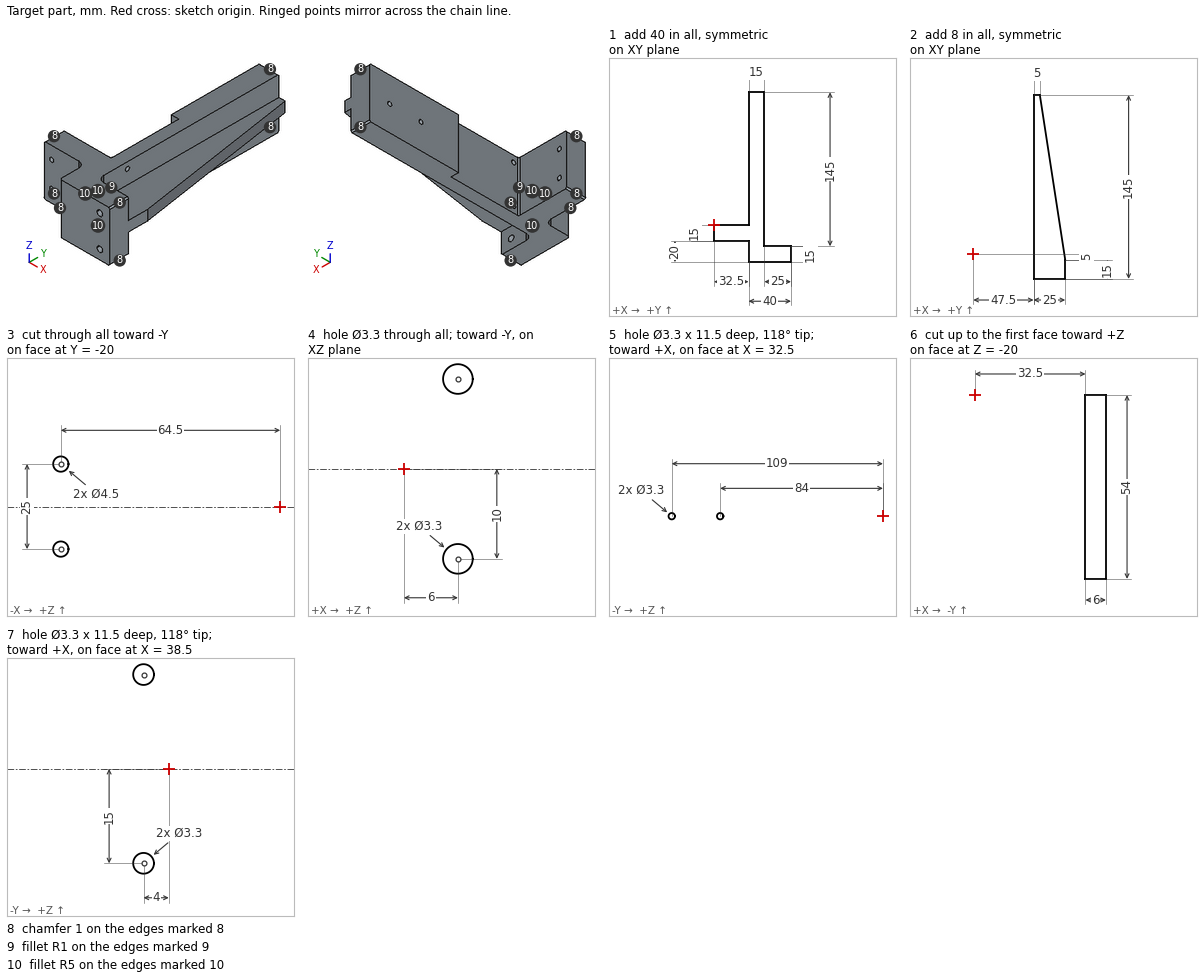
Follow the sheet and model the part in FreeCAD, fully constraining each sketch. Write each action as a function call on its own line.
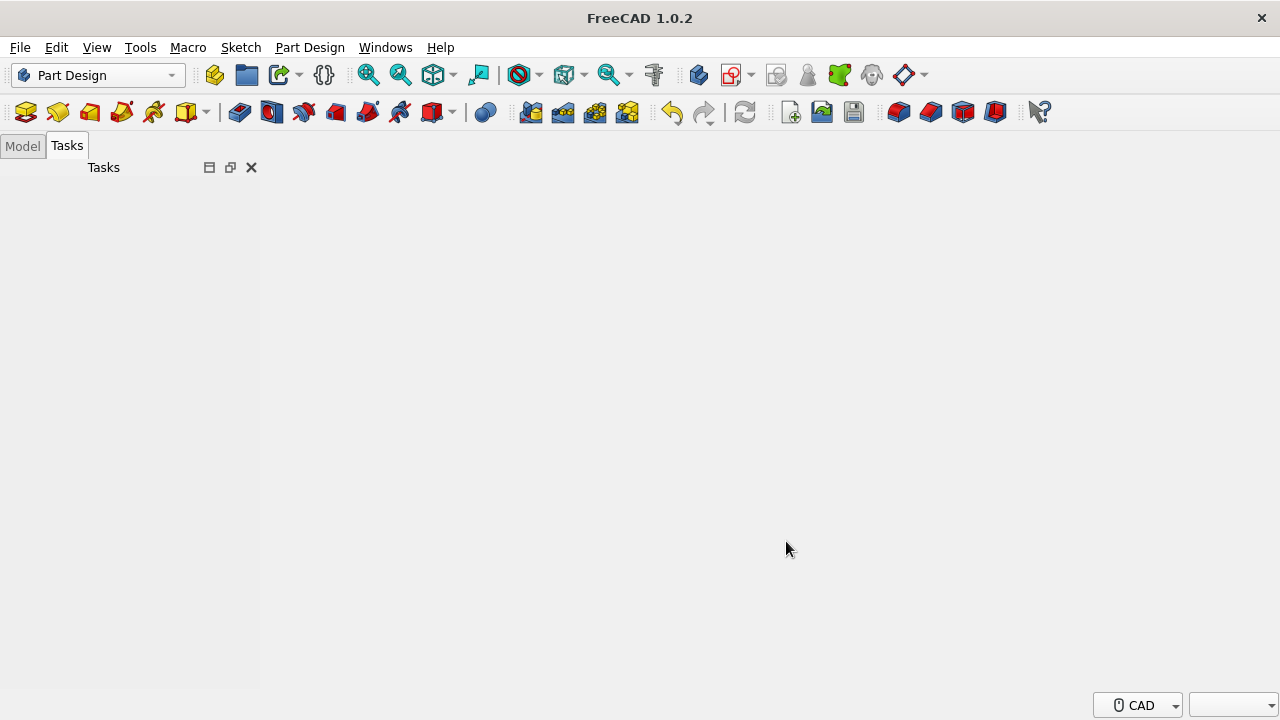
click(790, 112)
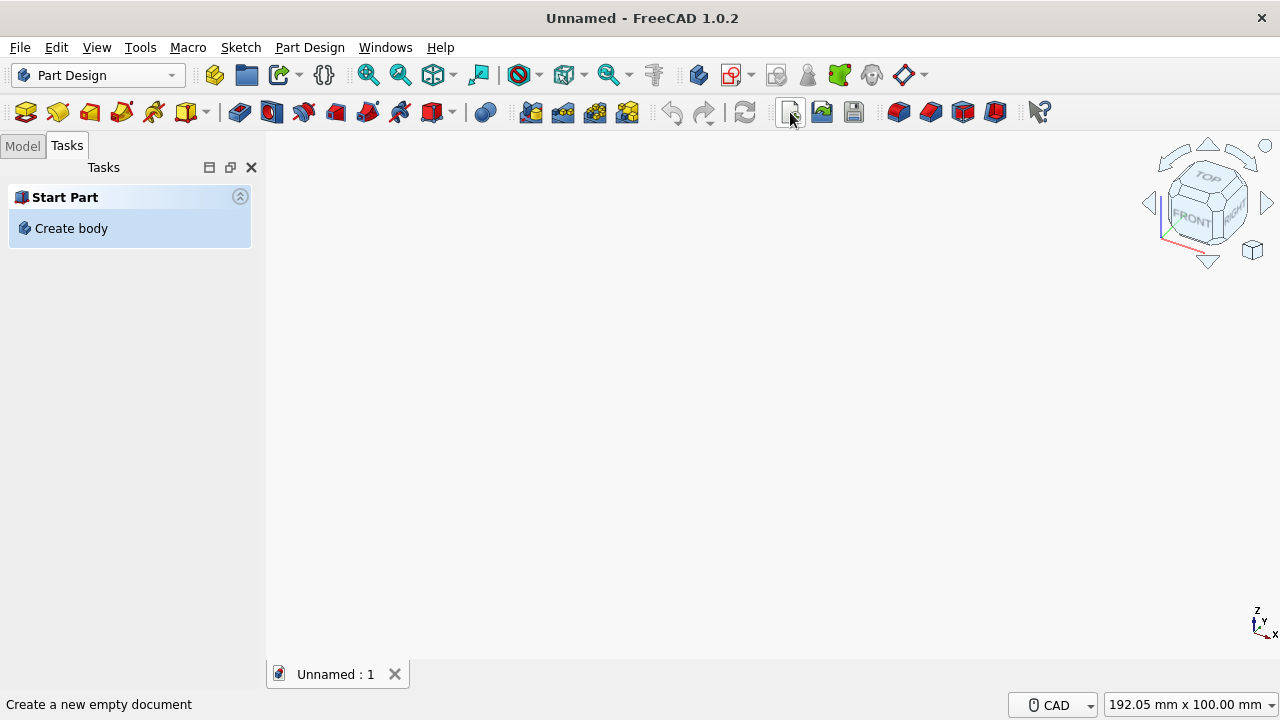
click(732, 76)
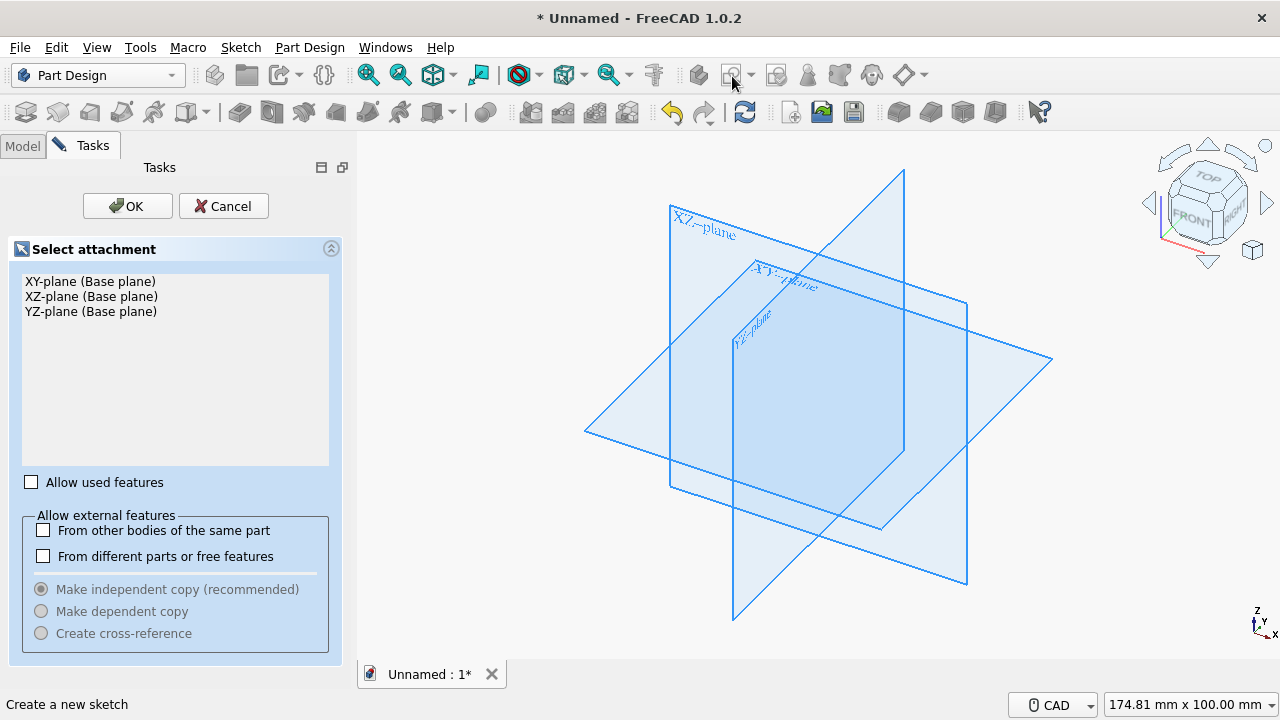
click(82, 282)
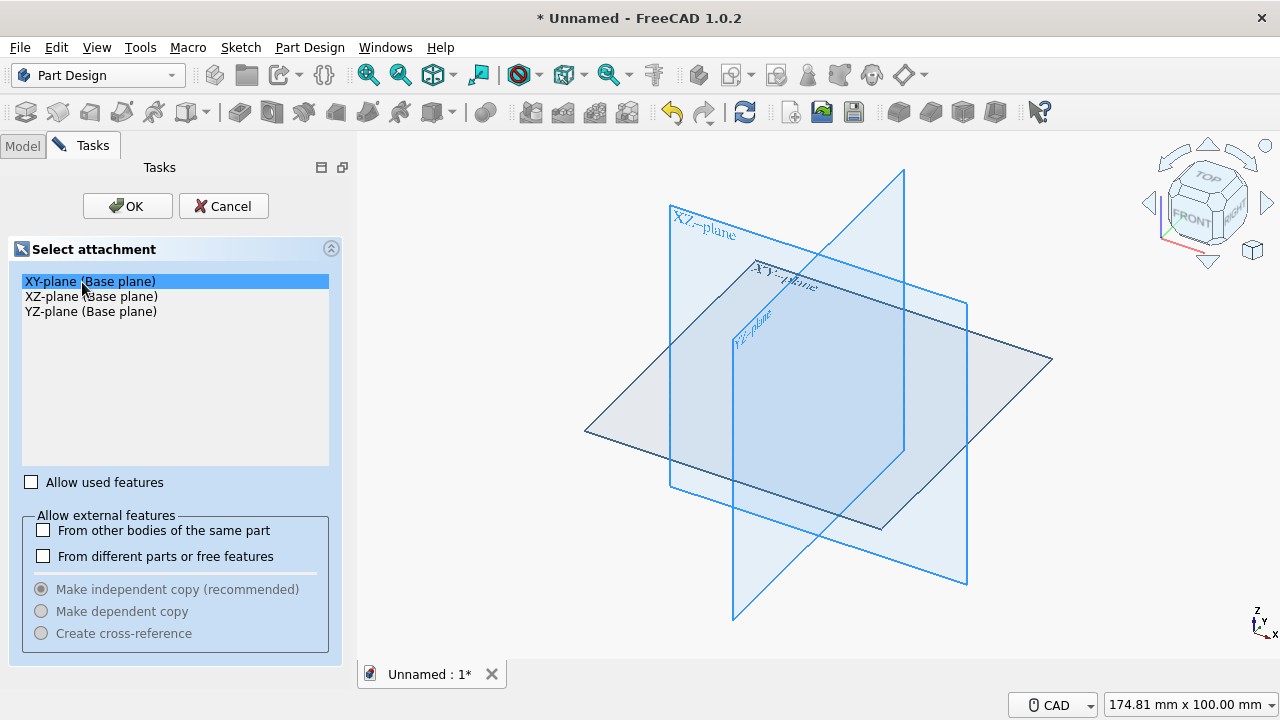
click(128, 206)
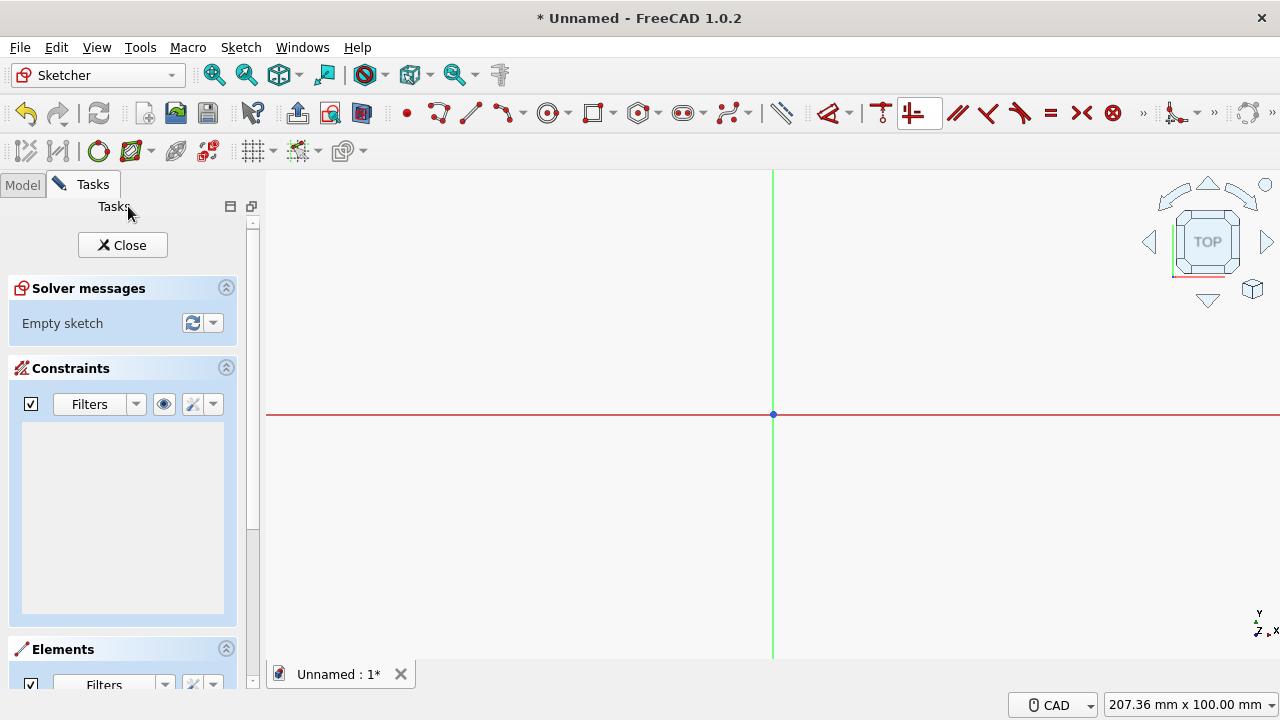
scroll(561, 543, down, 5)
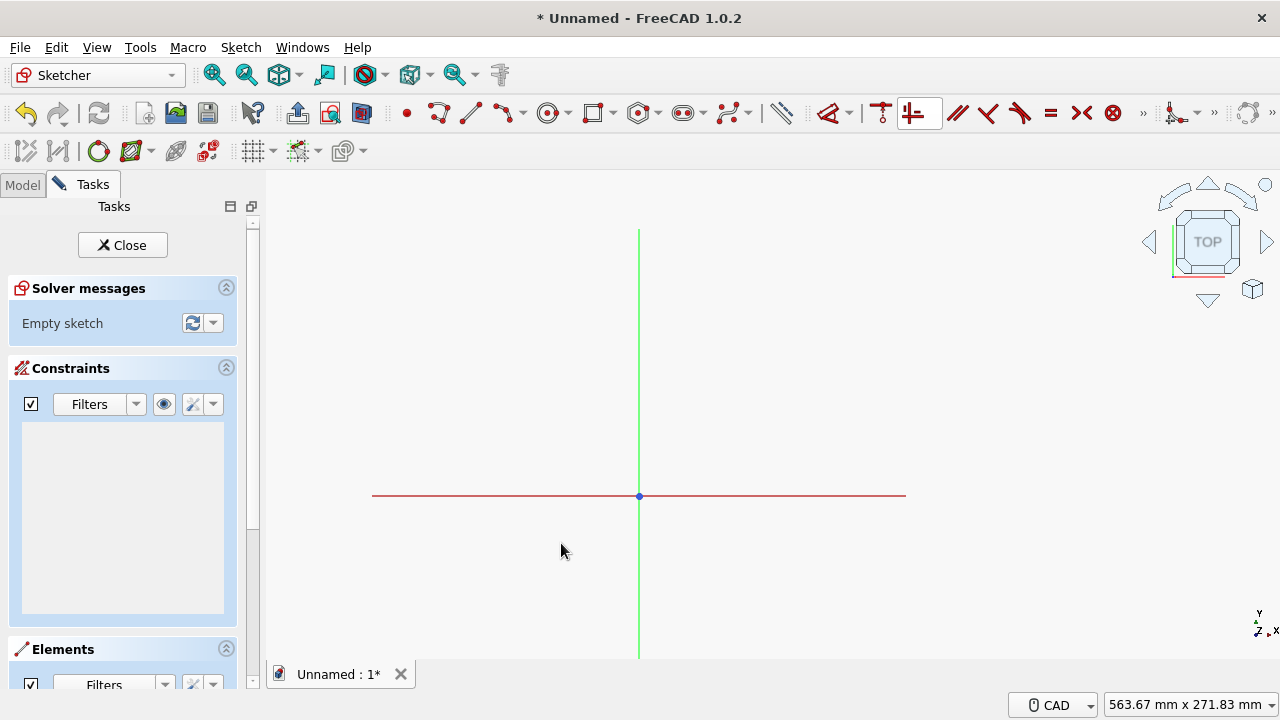
click(440, 114)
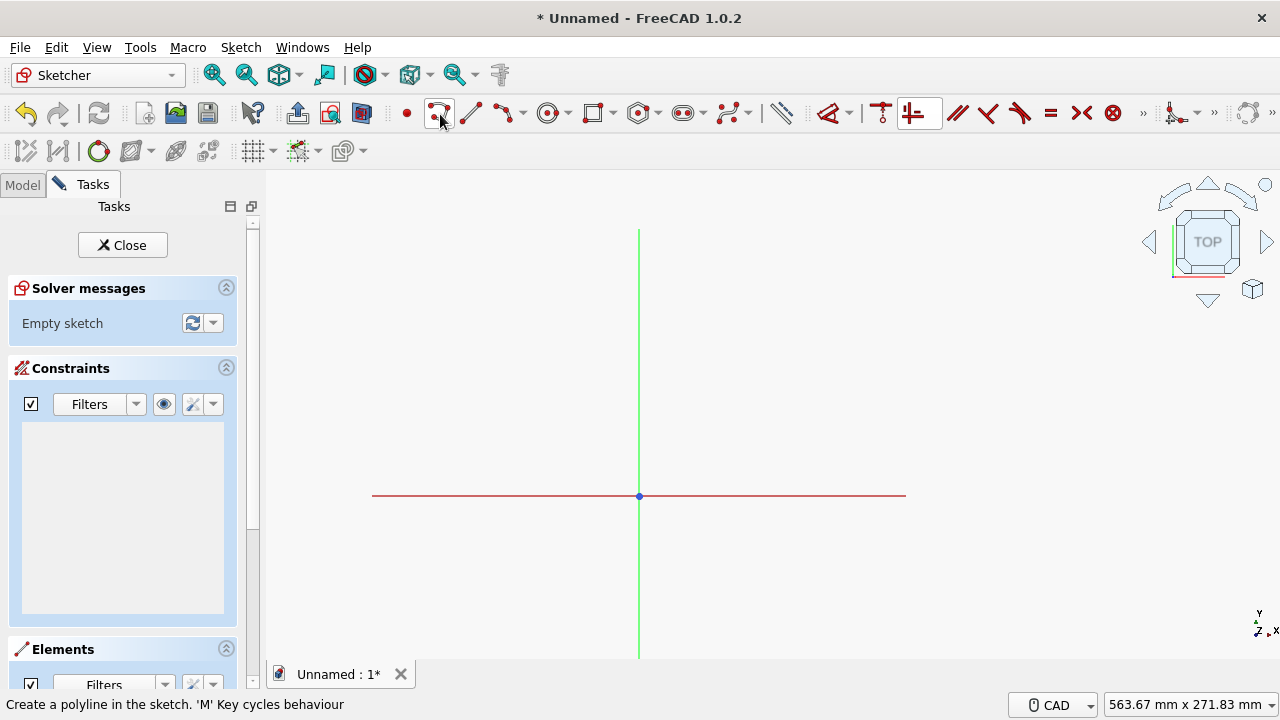
click(639, 496)
click(648, 523)
click(698, 523)
click(698, 559)
click(770, 559)
click(770, 532)
click(725, 532)
click(725, 271)
click(698, 271)
click(698, 487)
click(639, 496)
key(Escape)
key(Escape)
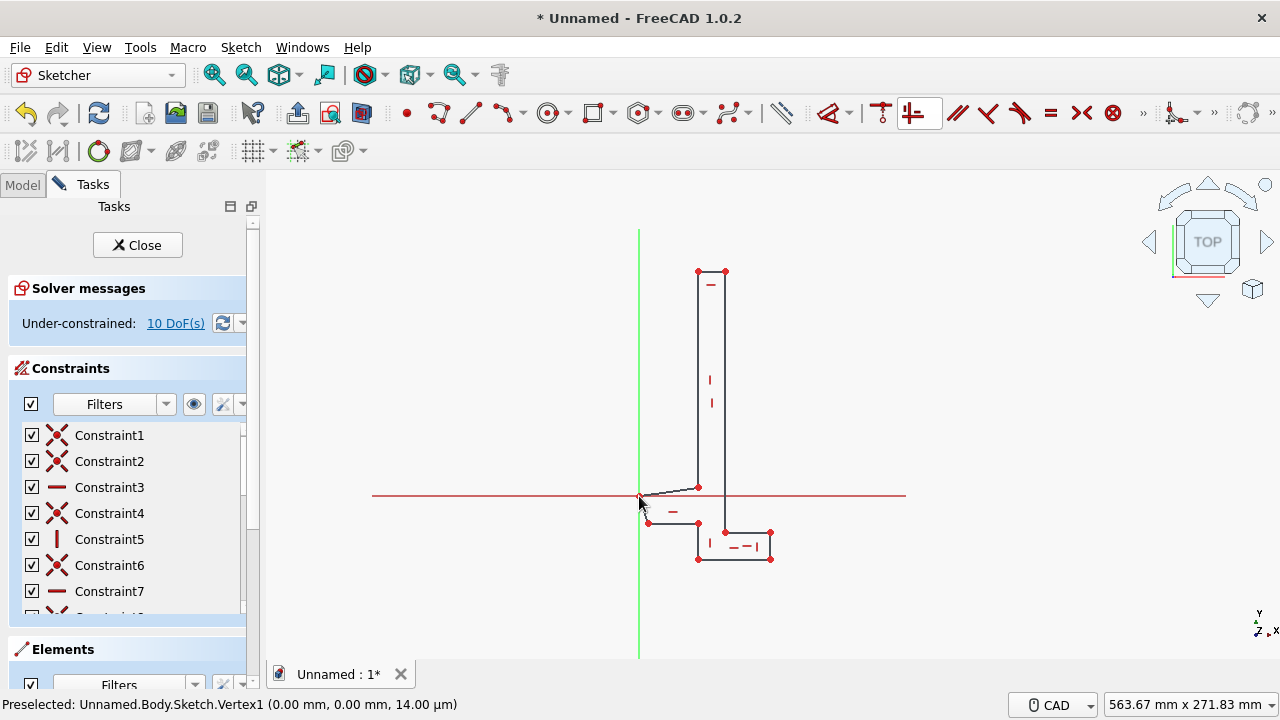
scroll(643, 507, up, 2)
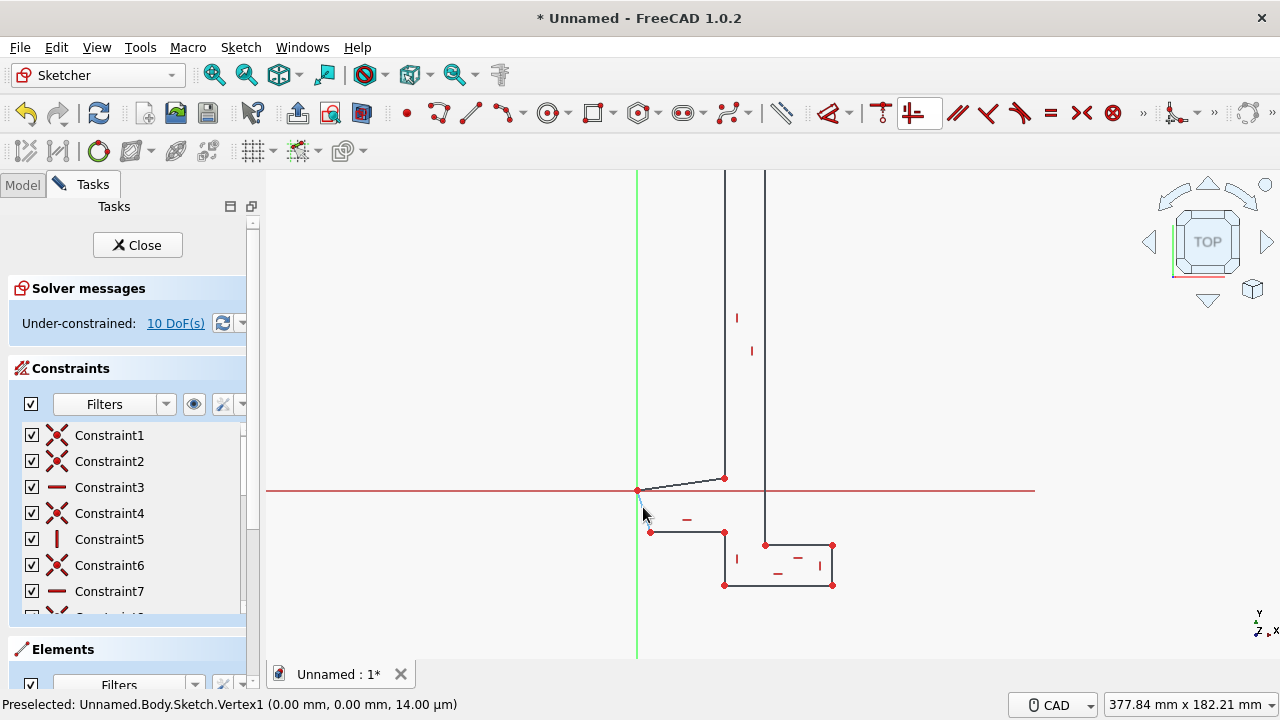
click(642, 507)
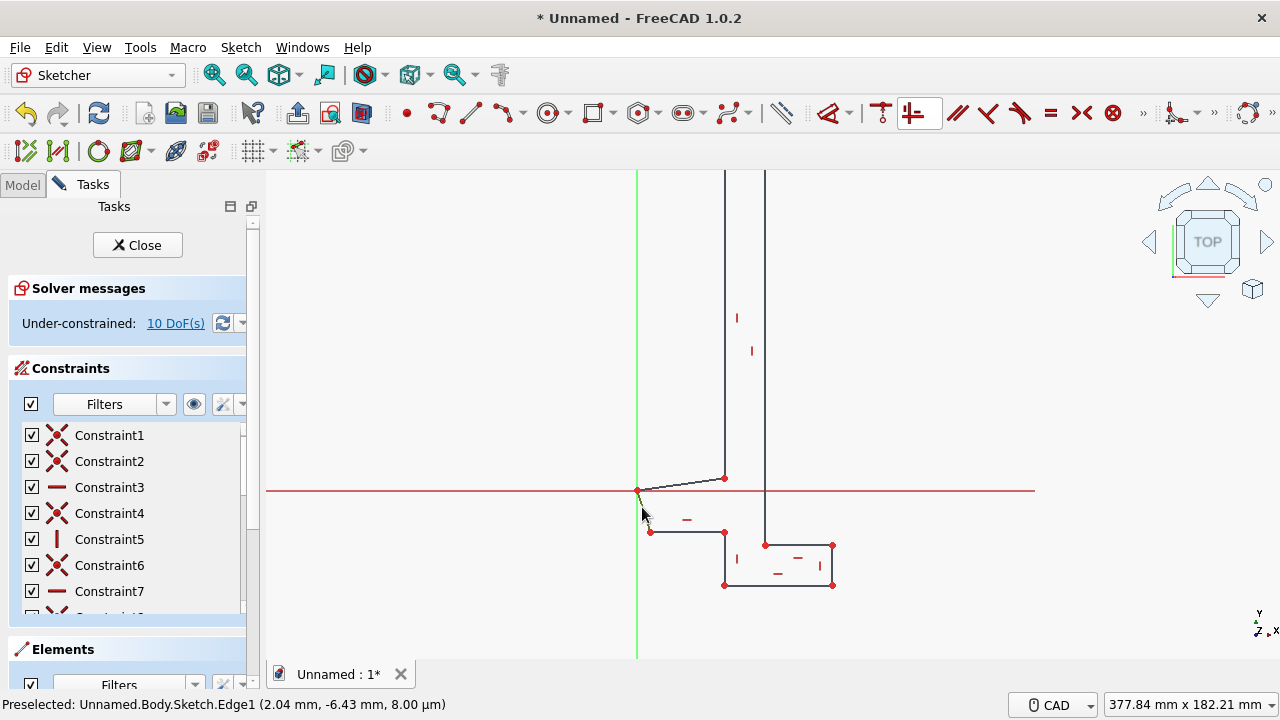
key(v)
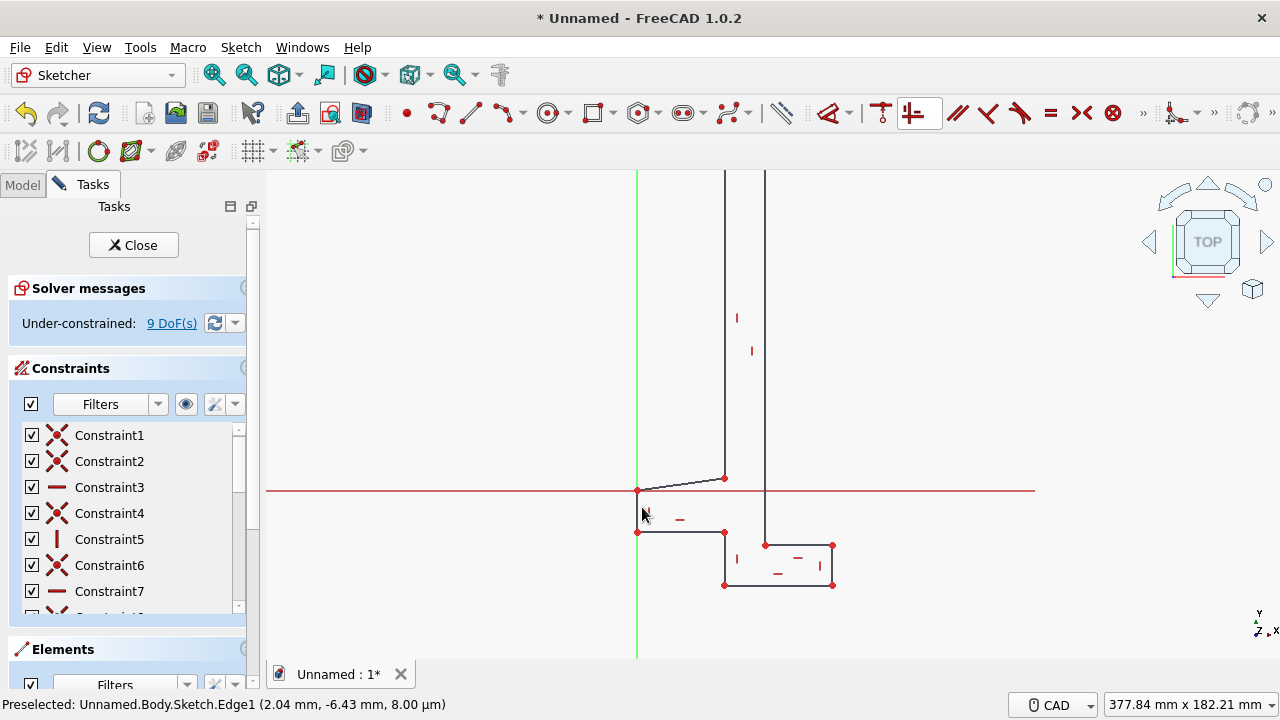
click(663, 487)